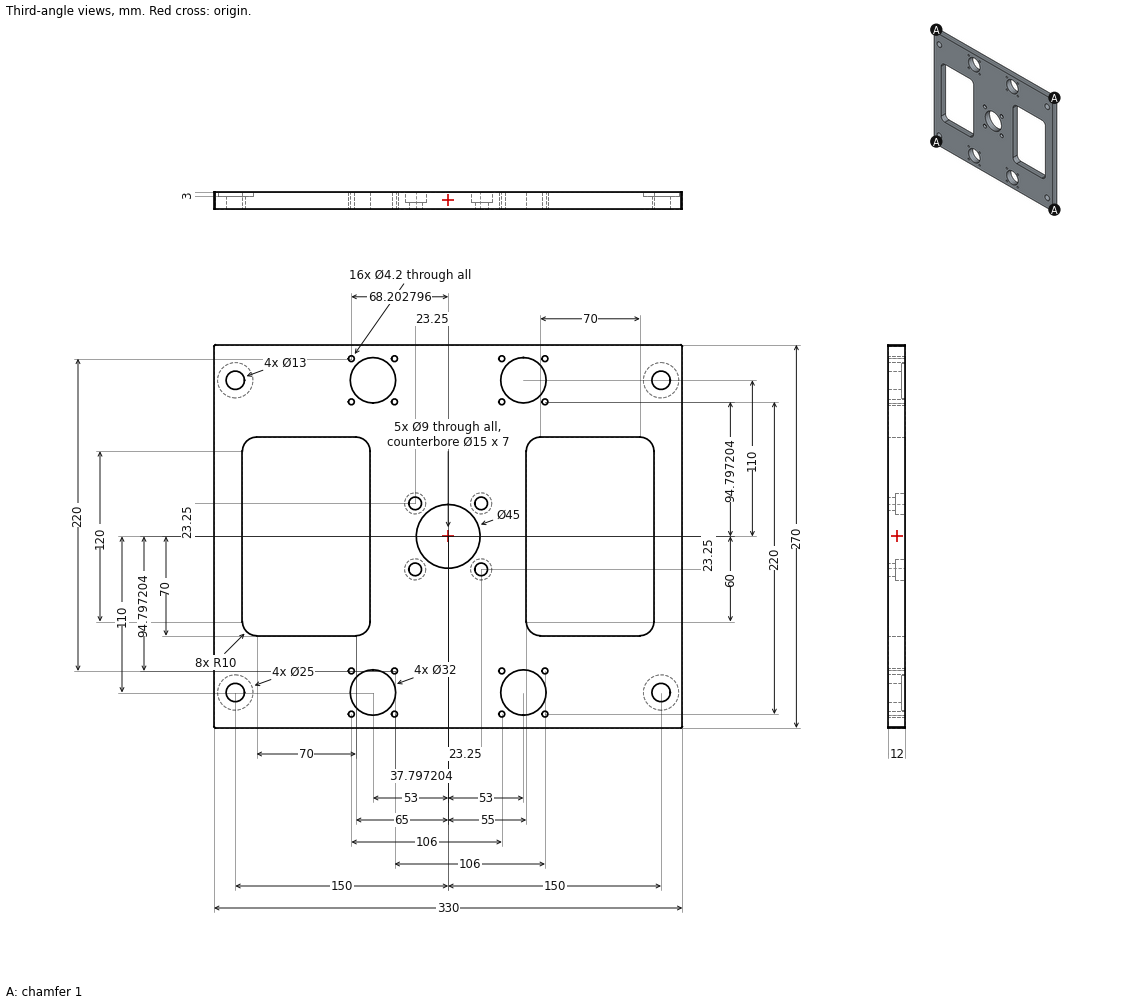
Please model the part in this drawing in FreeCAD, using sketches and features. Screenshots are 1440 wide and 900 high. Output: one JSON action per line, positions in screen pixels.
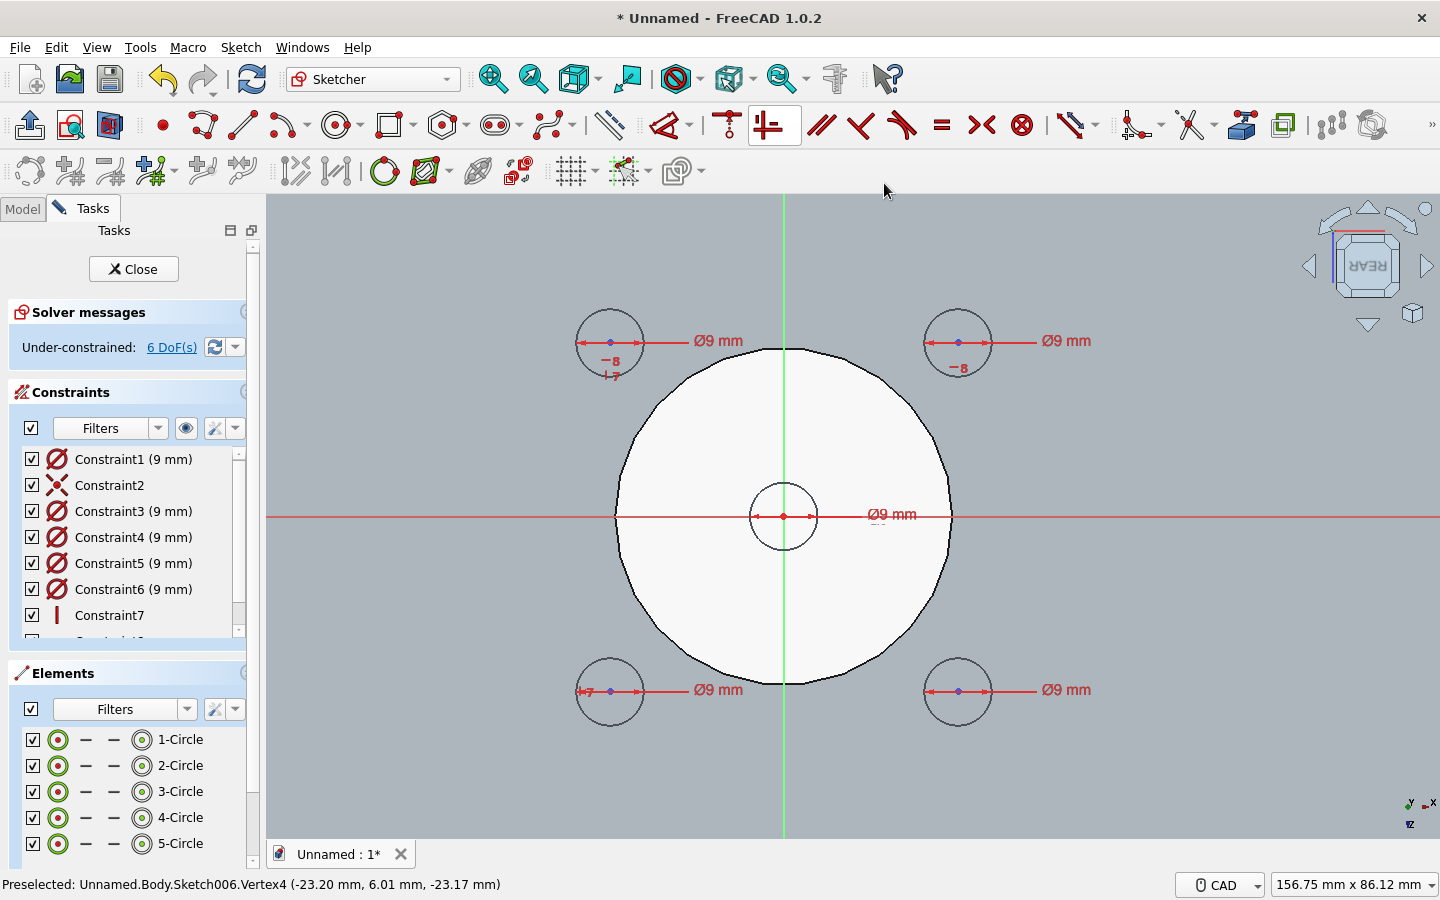
{"action": "left_click", "coordinate": [958, 343]}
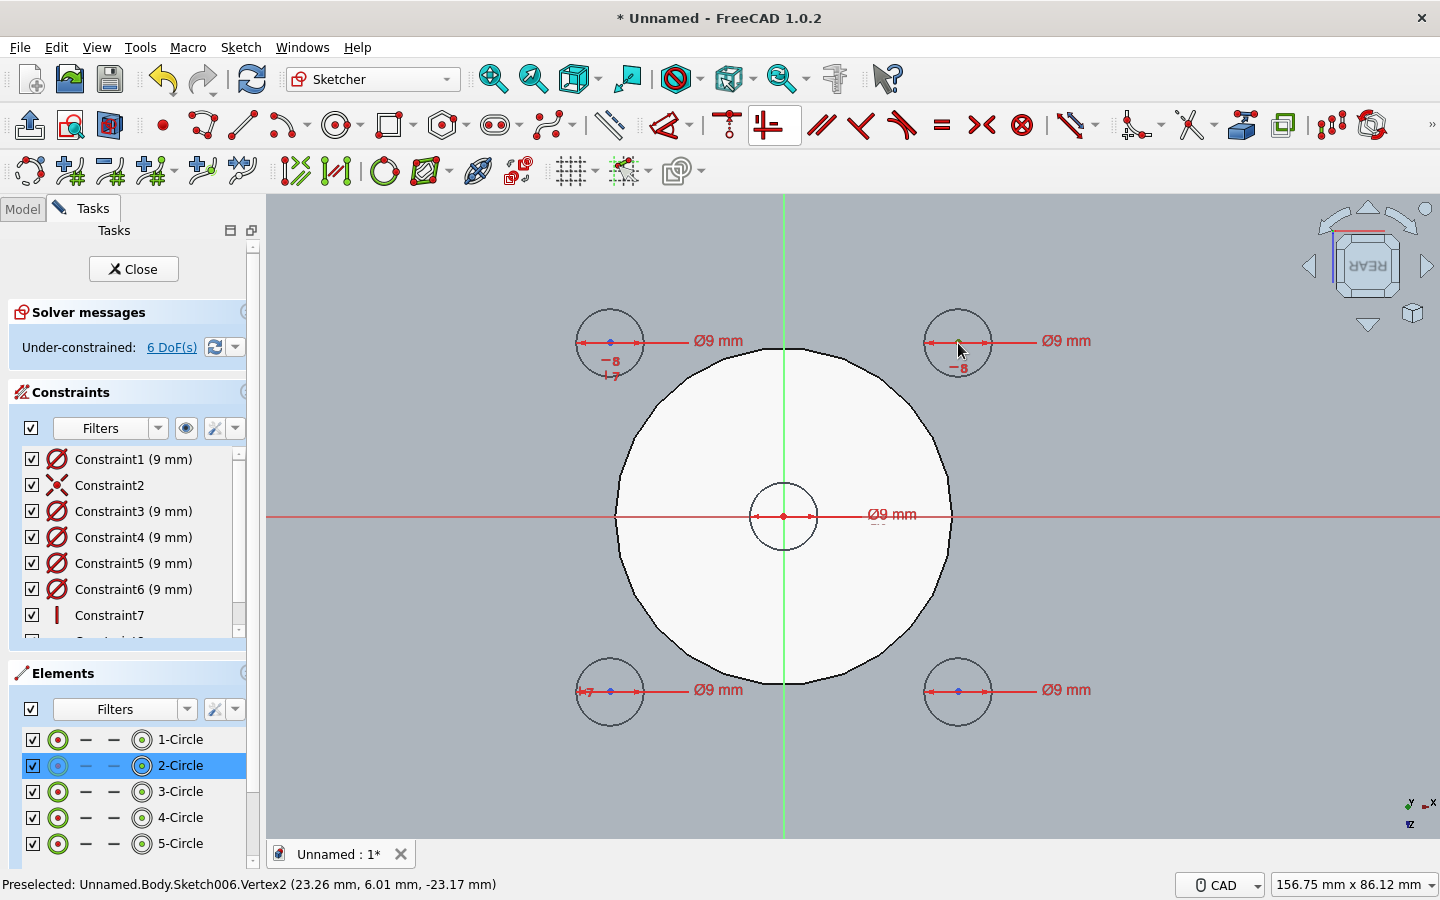
{"action": "left_click", "coordinate": [958, 692]}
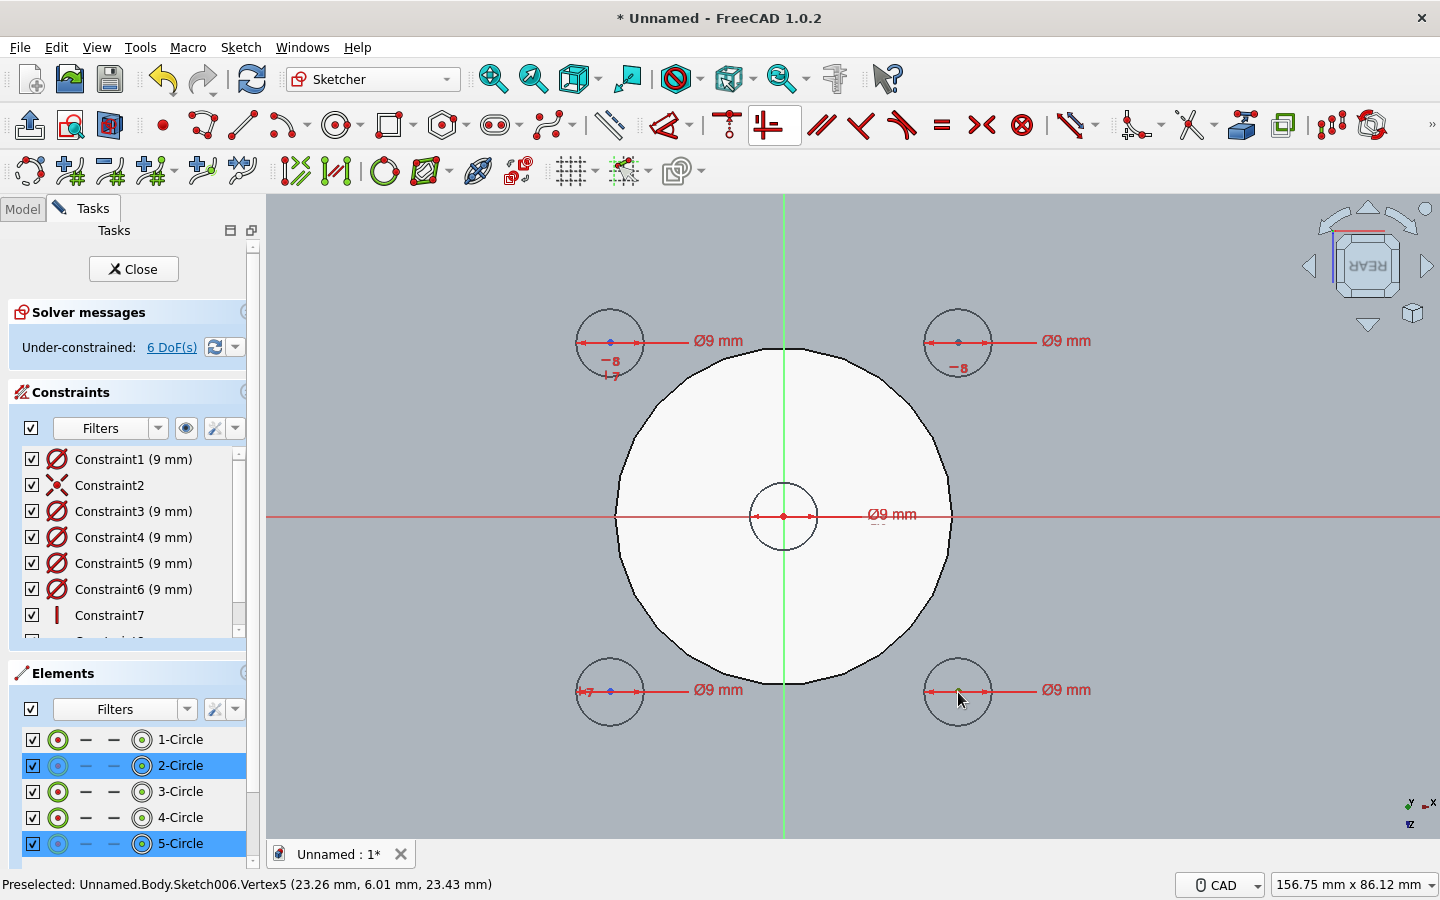
{"action": "left_click", "coordinate": [796, 126]}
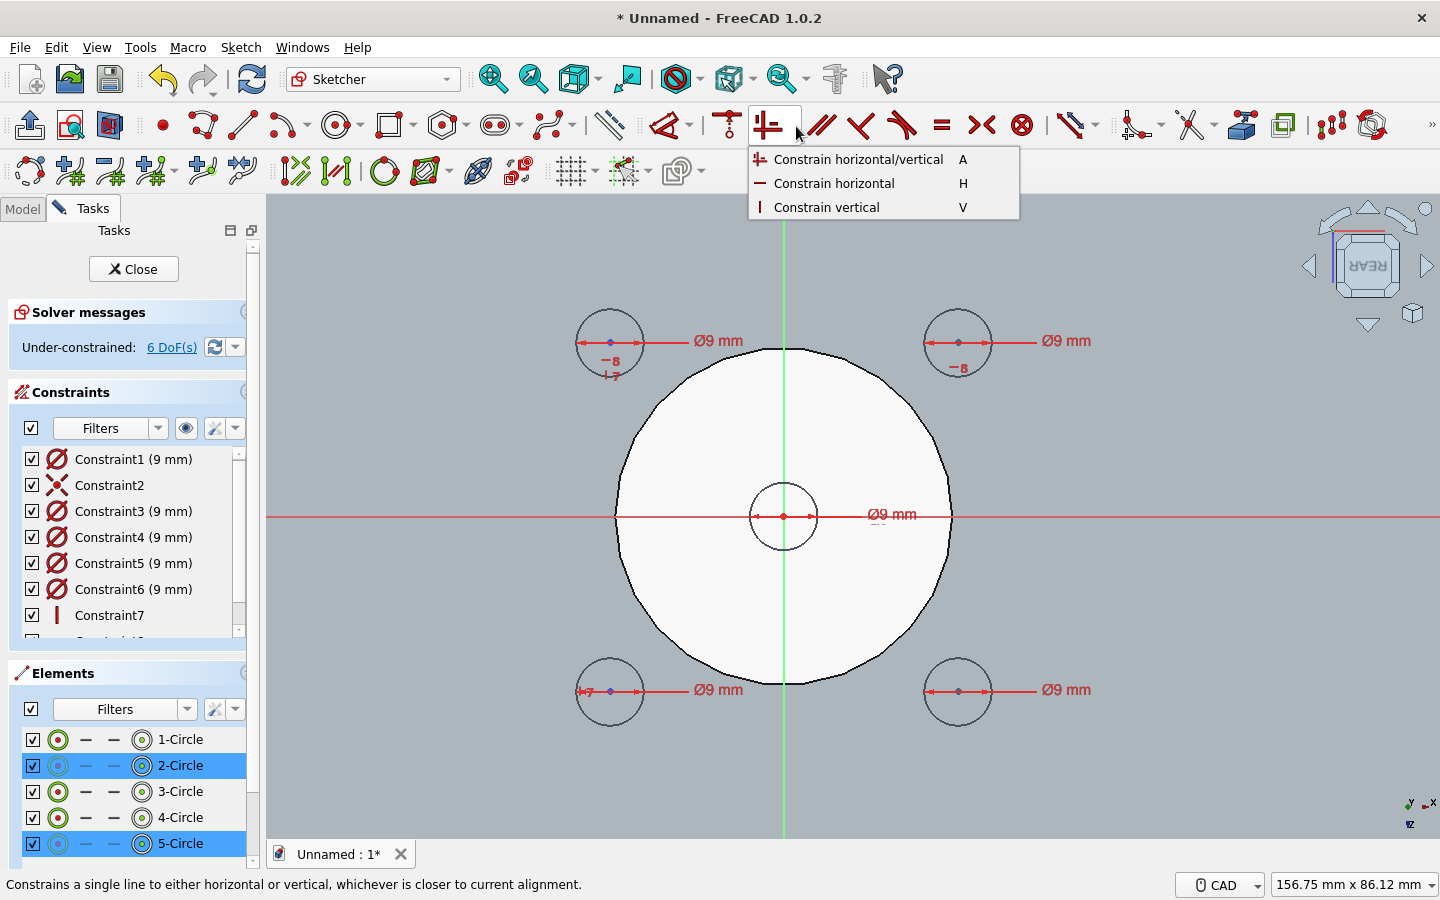
{"action": "left_click", "coordinate": [884, 207]}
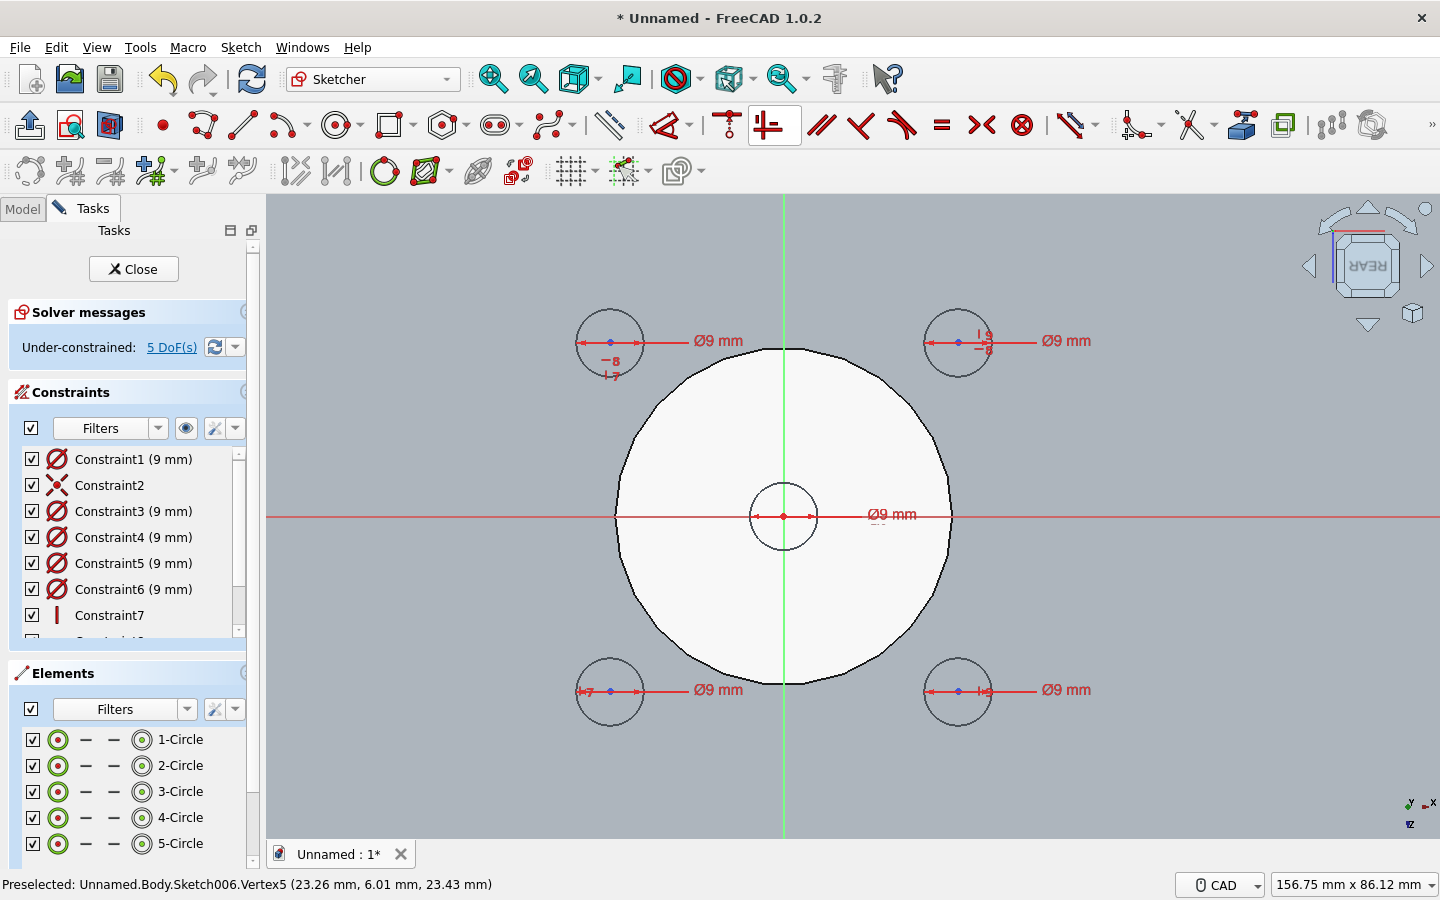
{"action": "left_click", "coordinate": [610, 692]}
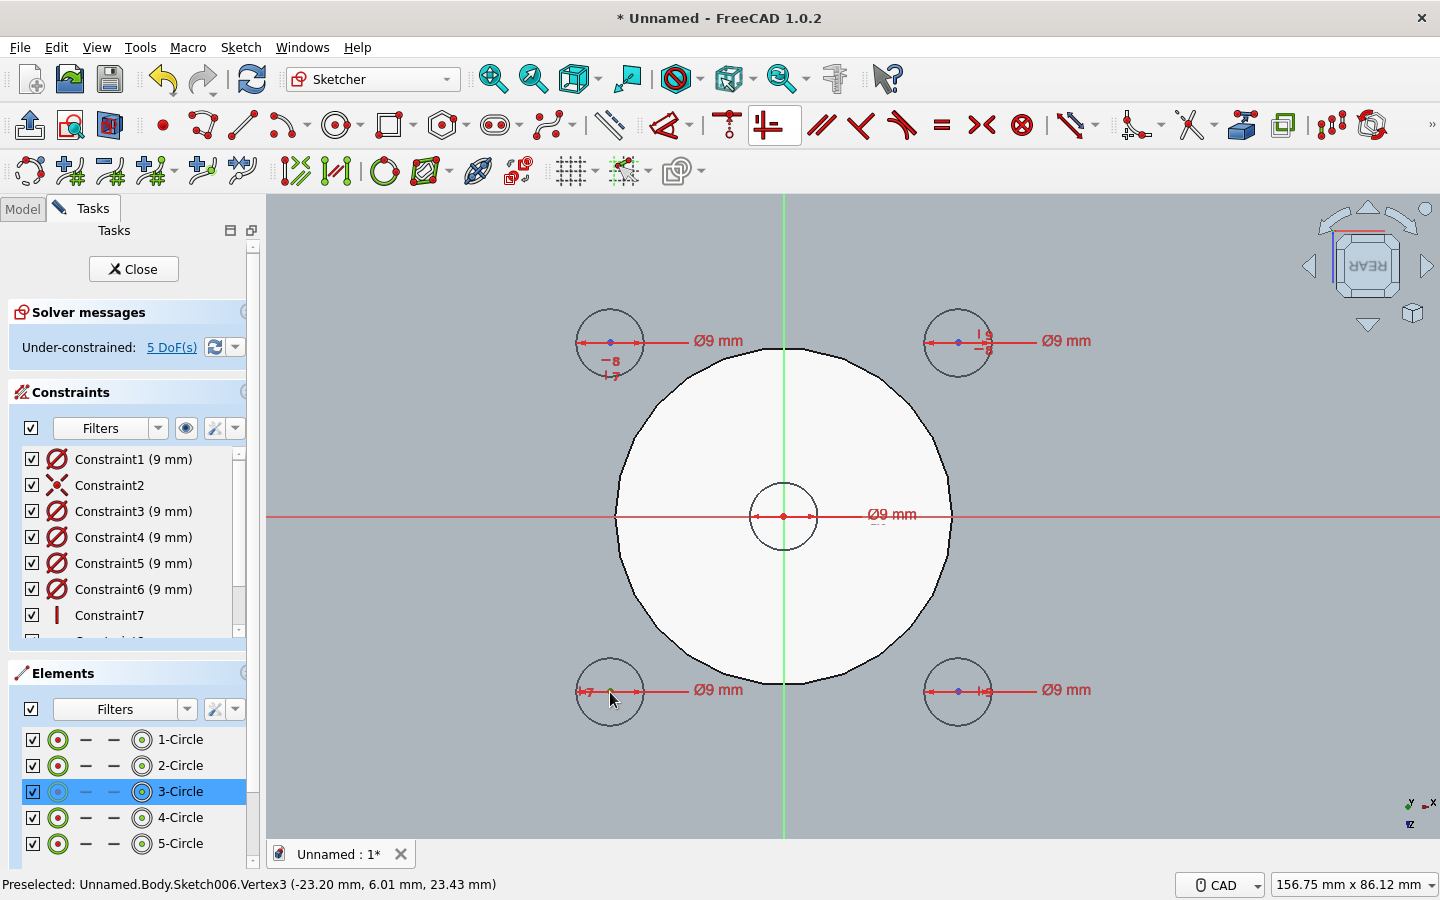
{"action": "left_click", "coordinate": [958, 692]}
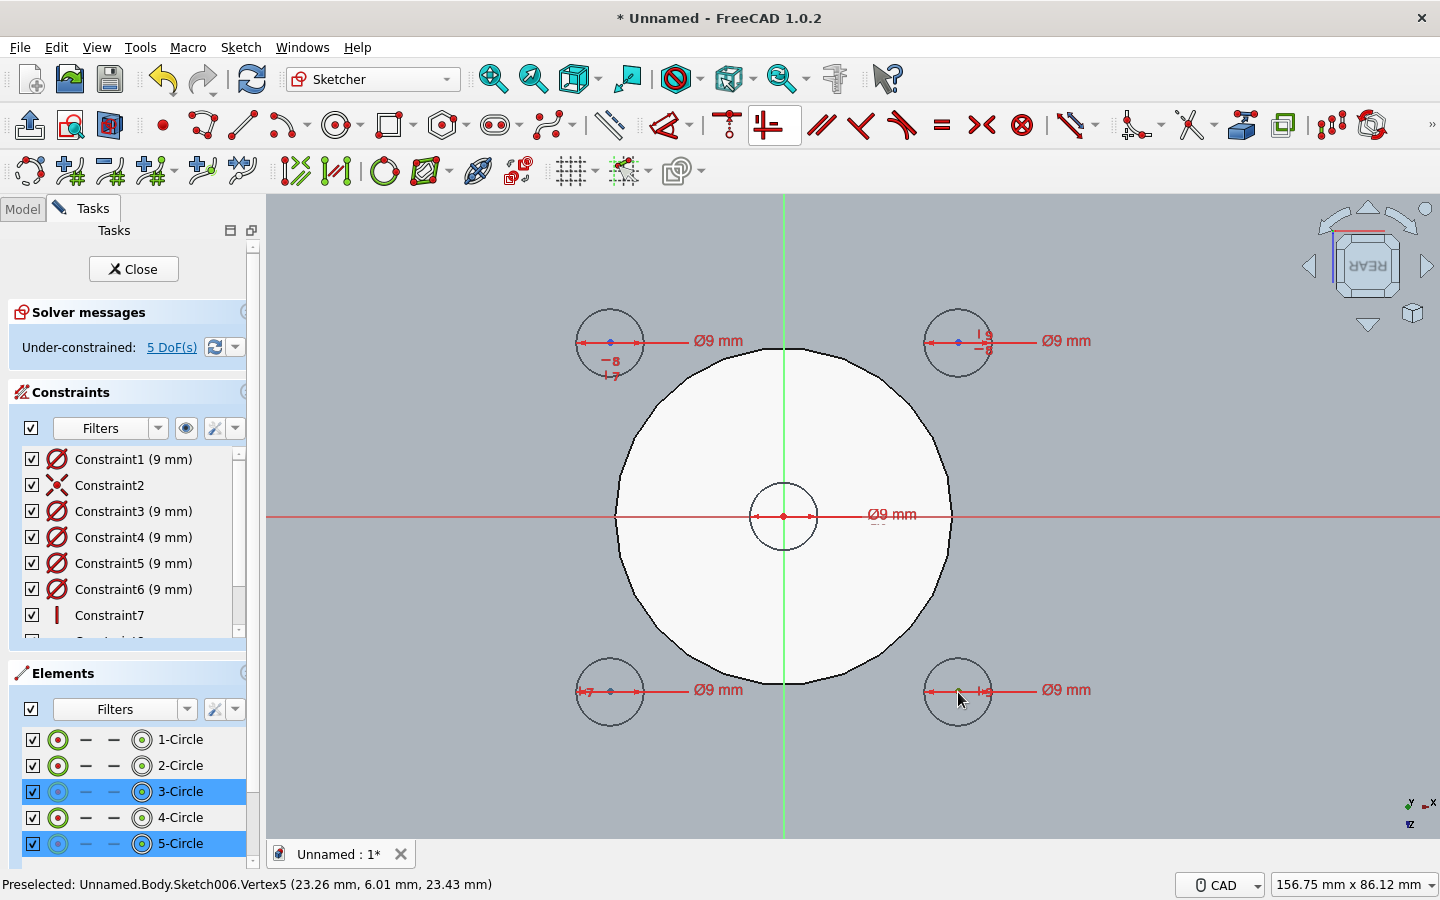
{"action": "key", "text": "h"}